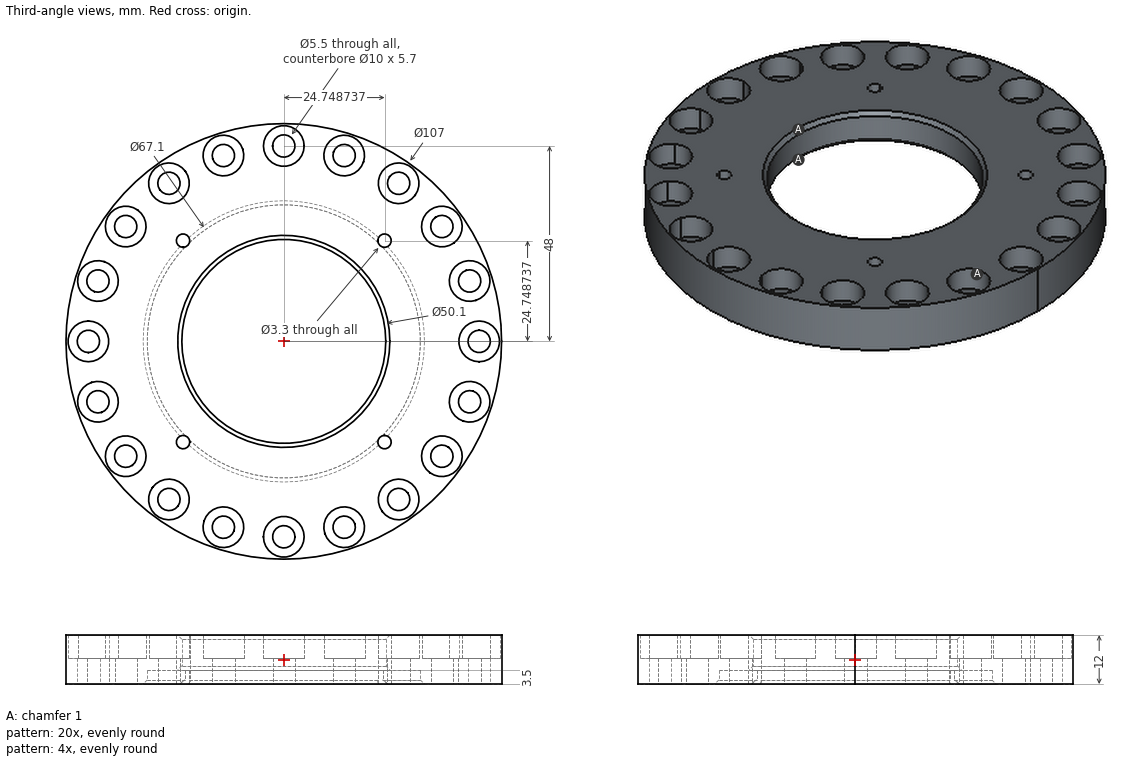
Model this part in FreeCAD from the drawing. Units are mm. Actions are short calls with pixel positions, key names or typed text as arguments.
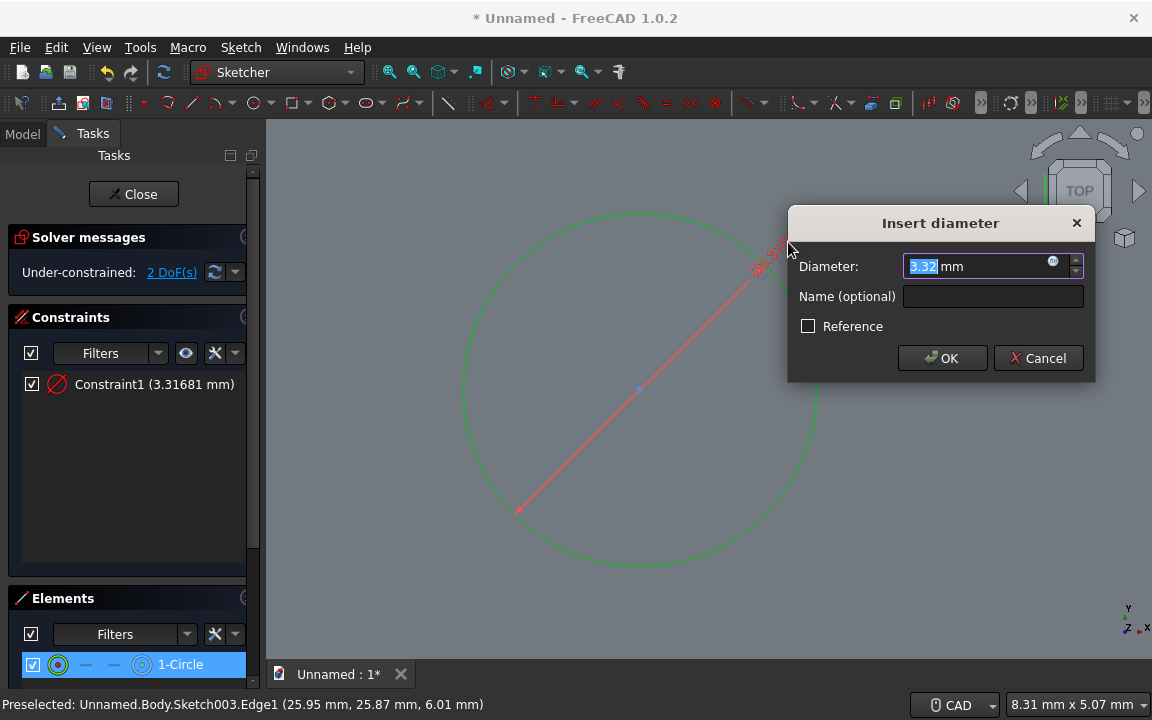
text(3.3)
key(Return)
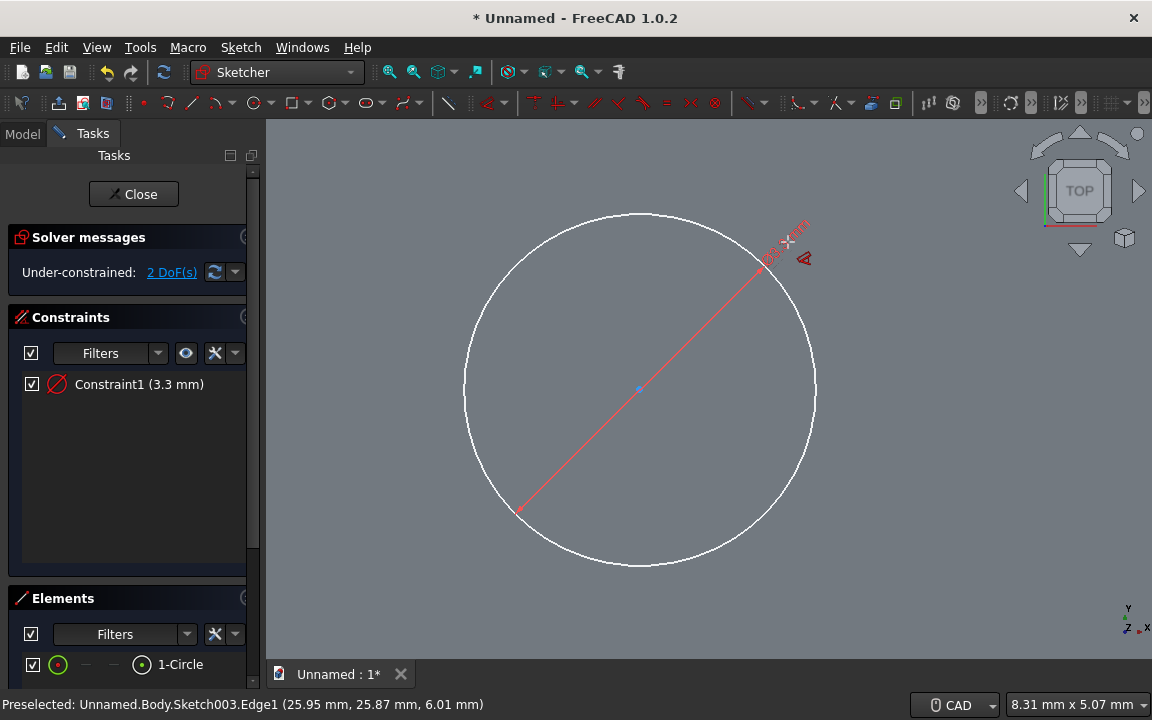
click(640, 390)
click(387, 356)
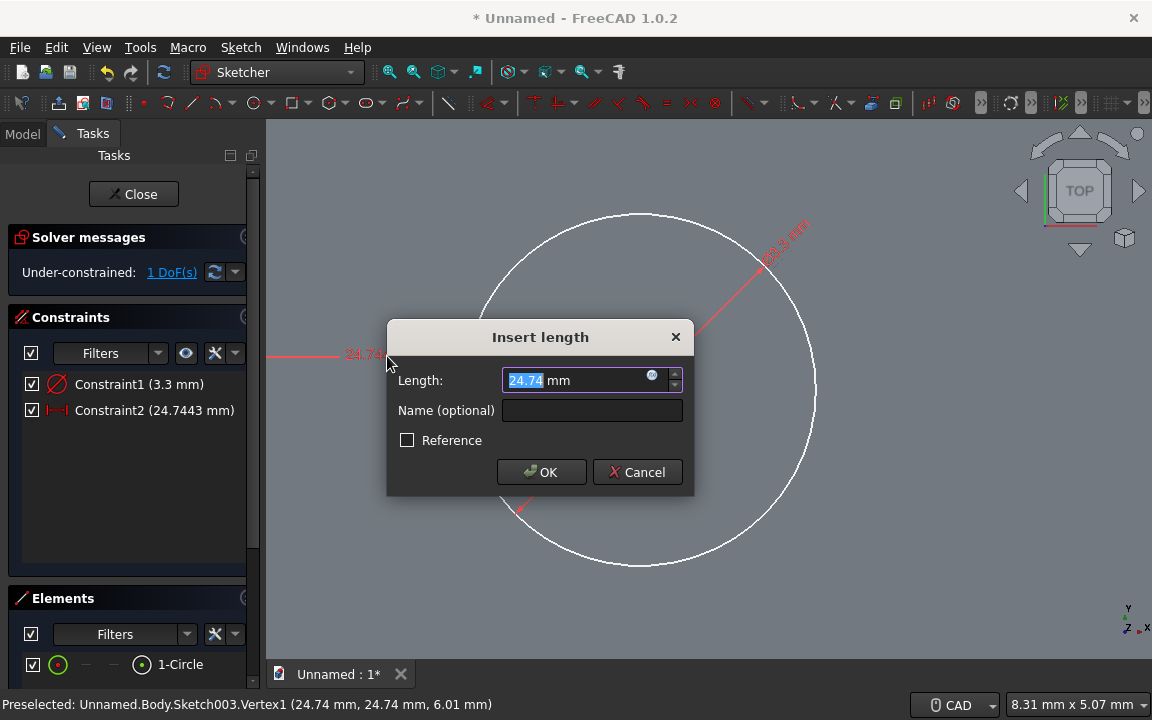
text(24.748737)
key(Return)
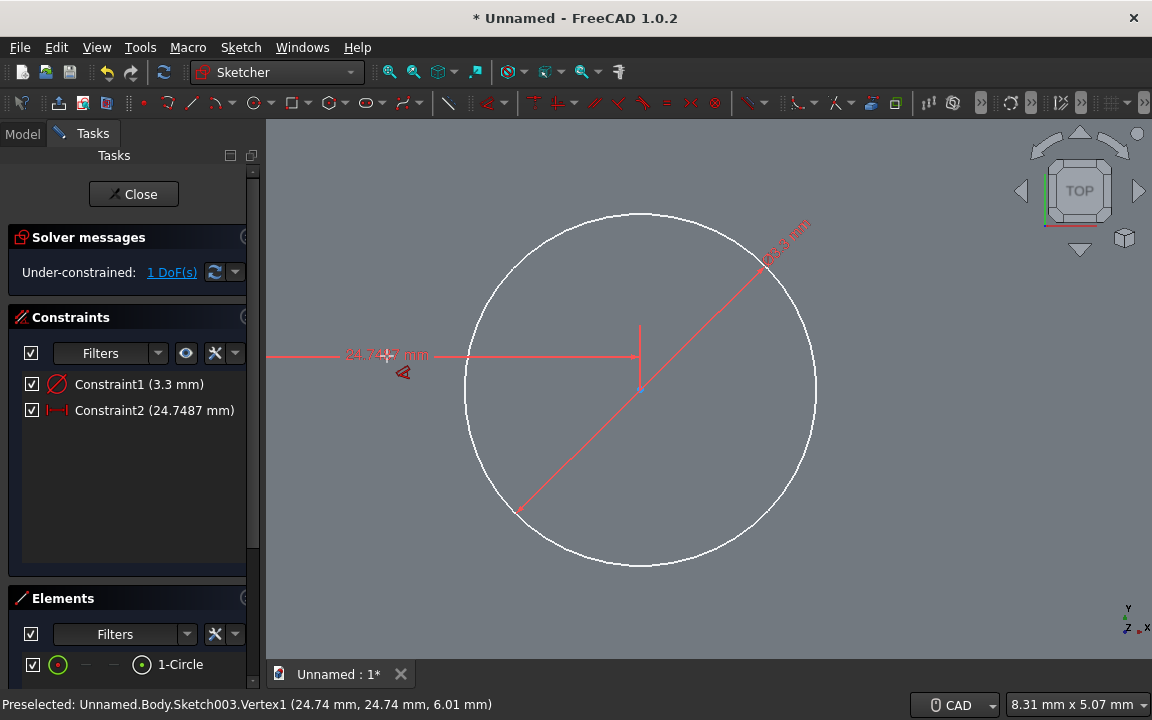
click(640, 390)
click(674, 511)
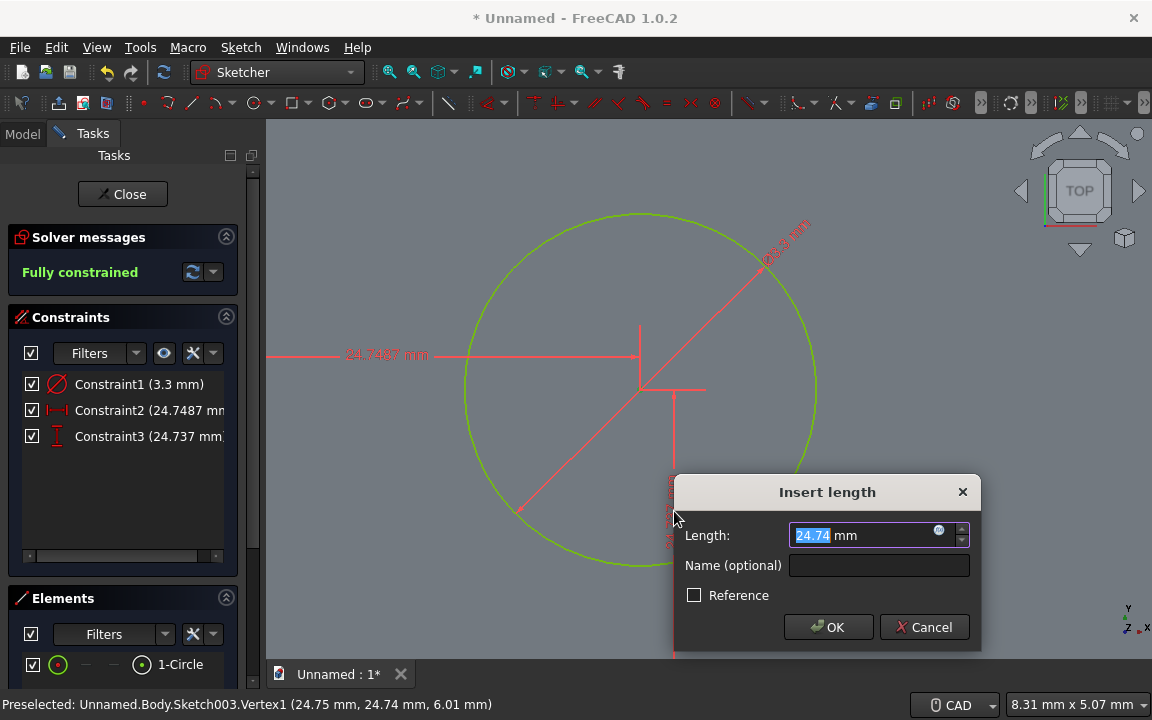
text(24.748737)
key(Return)
key(Escape)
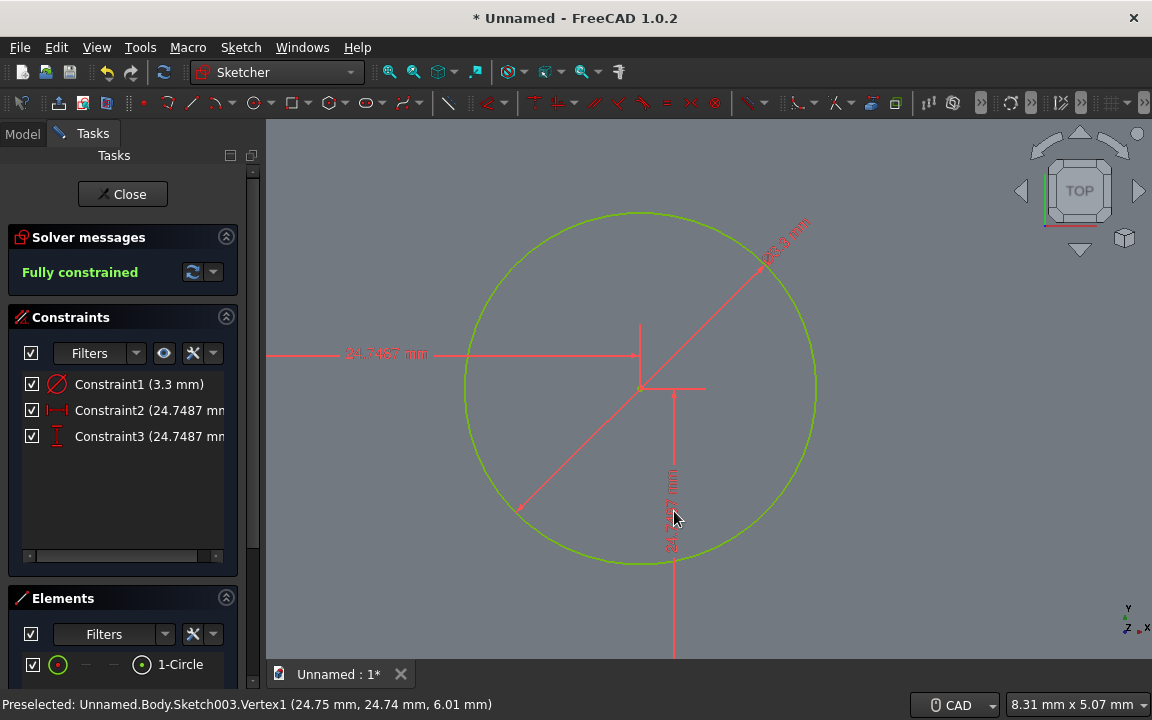
click(123, 194)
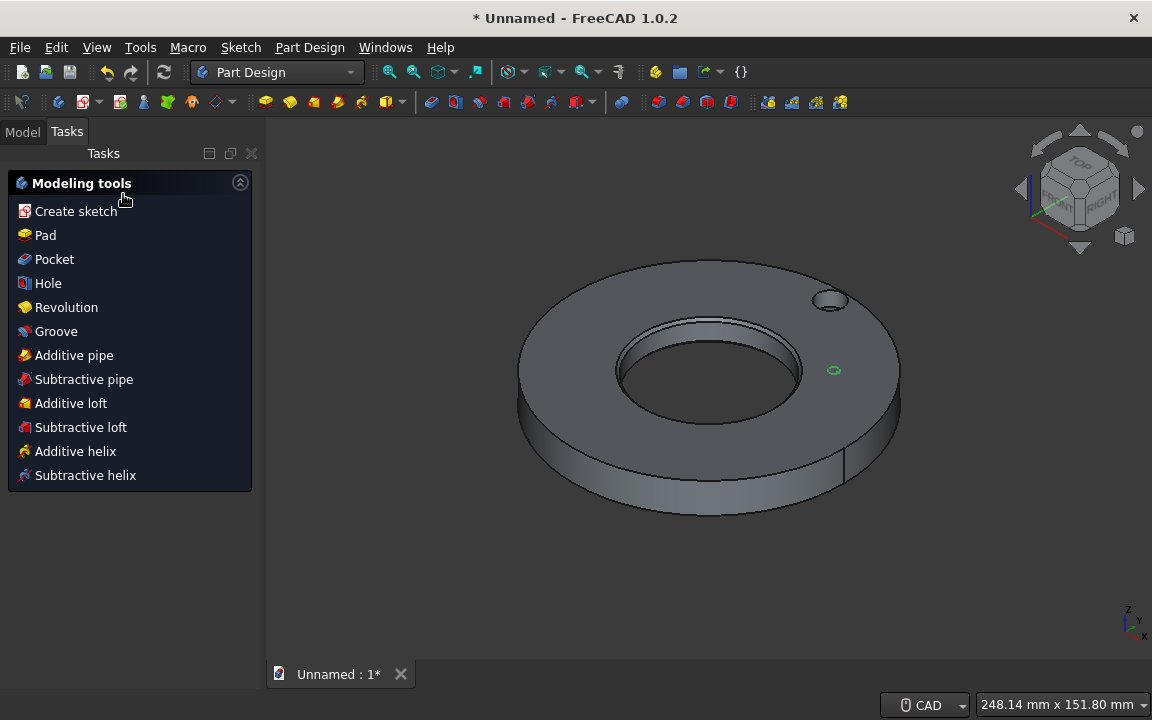
click(456, 102)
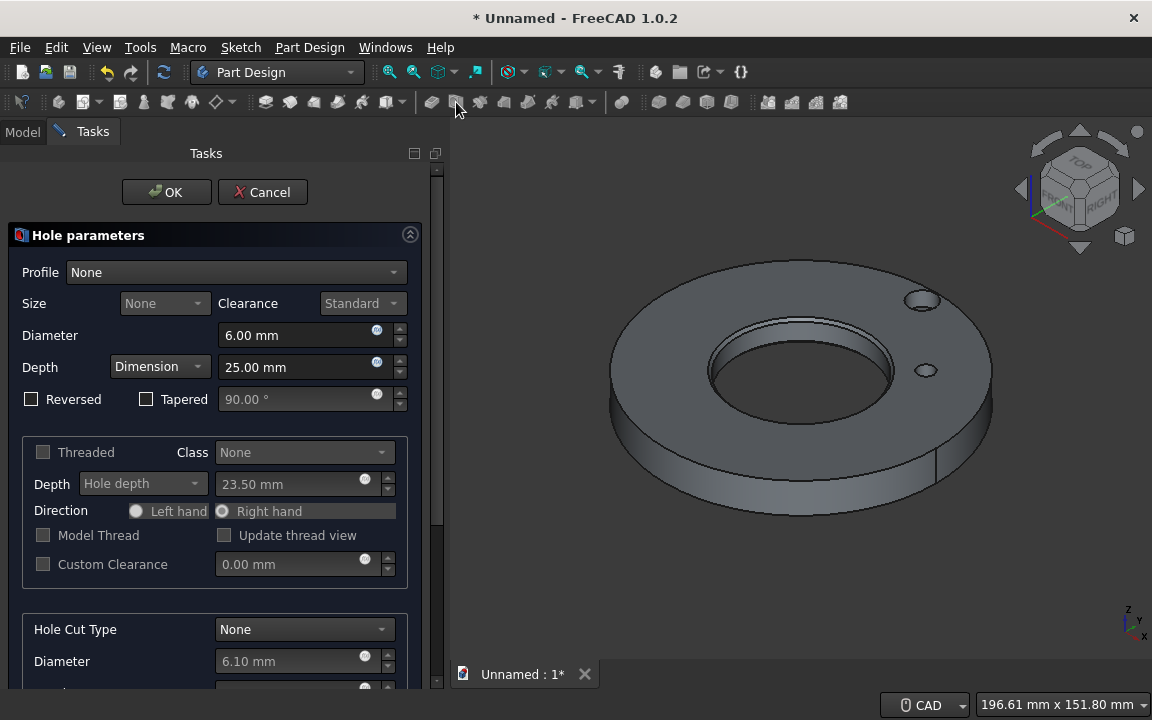
triple_click(305, 335)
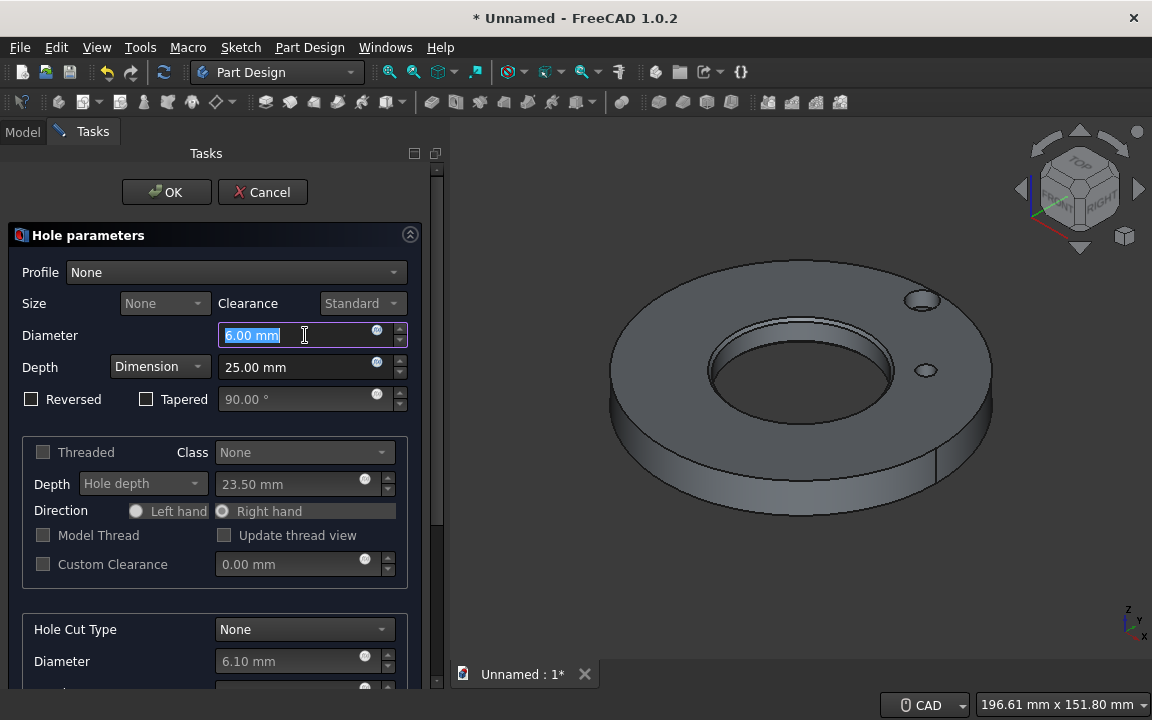
text(3.3)
key(Tab)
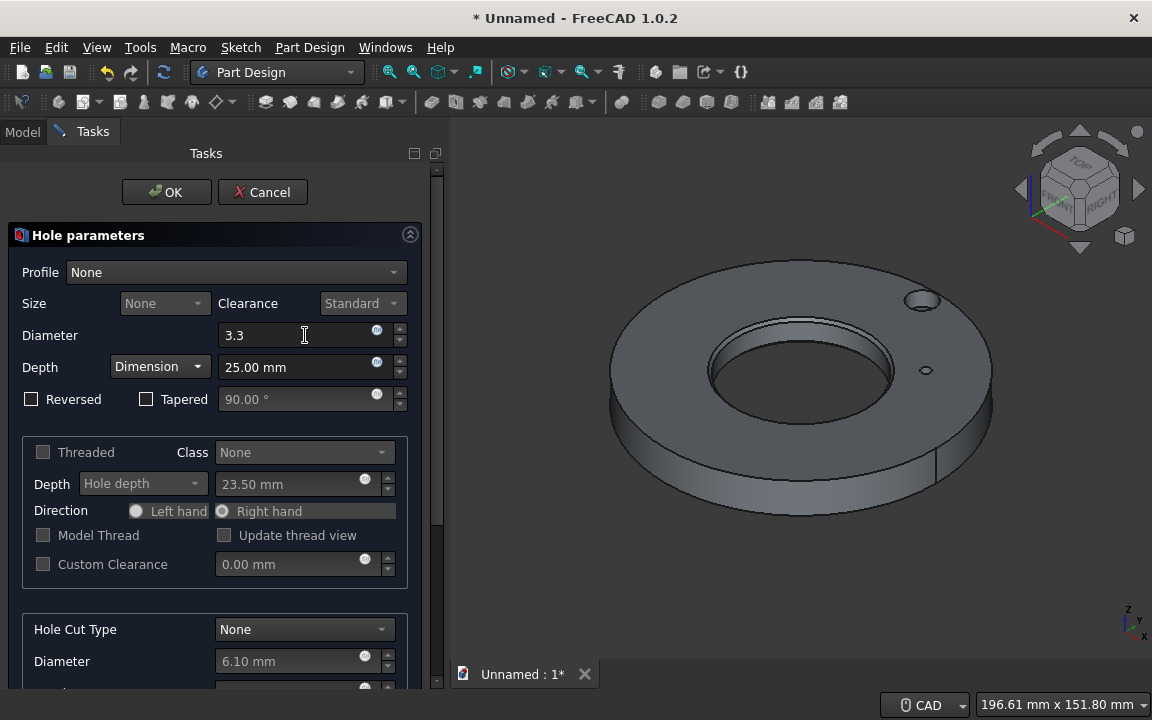
click(161, 366)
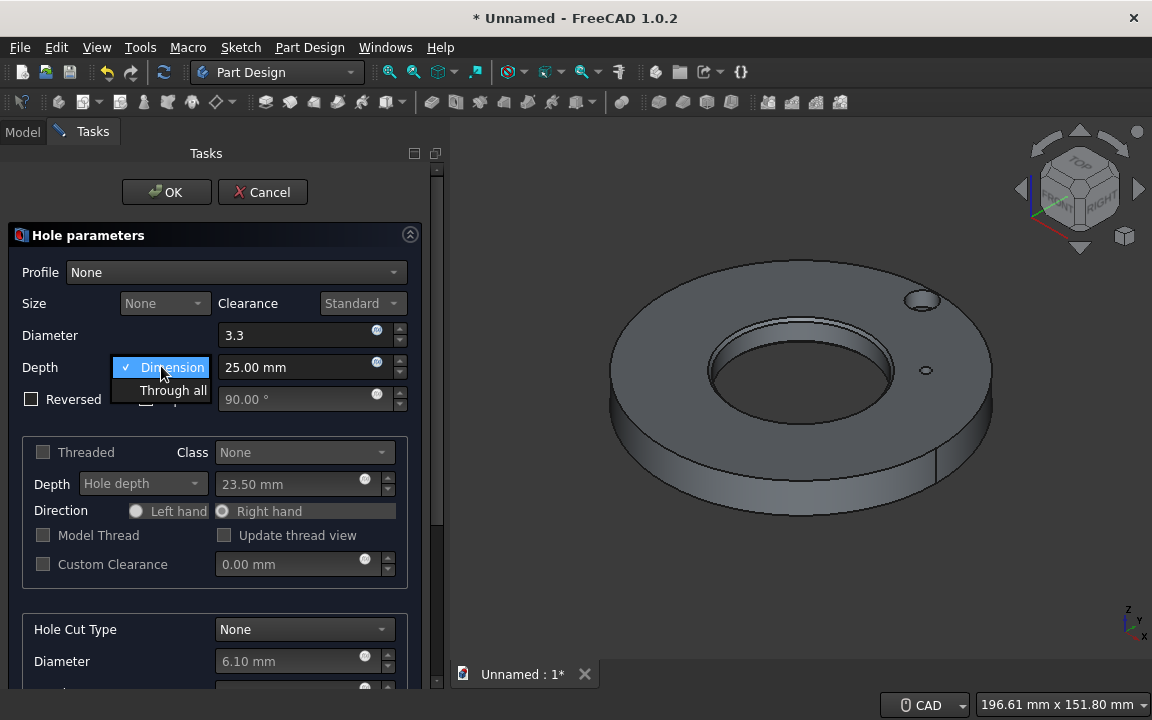
click(160, 390)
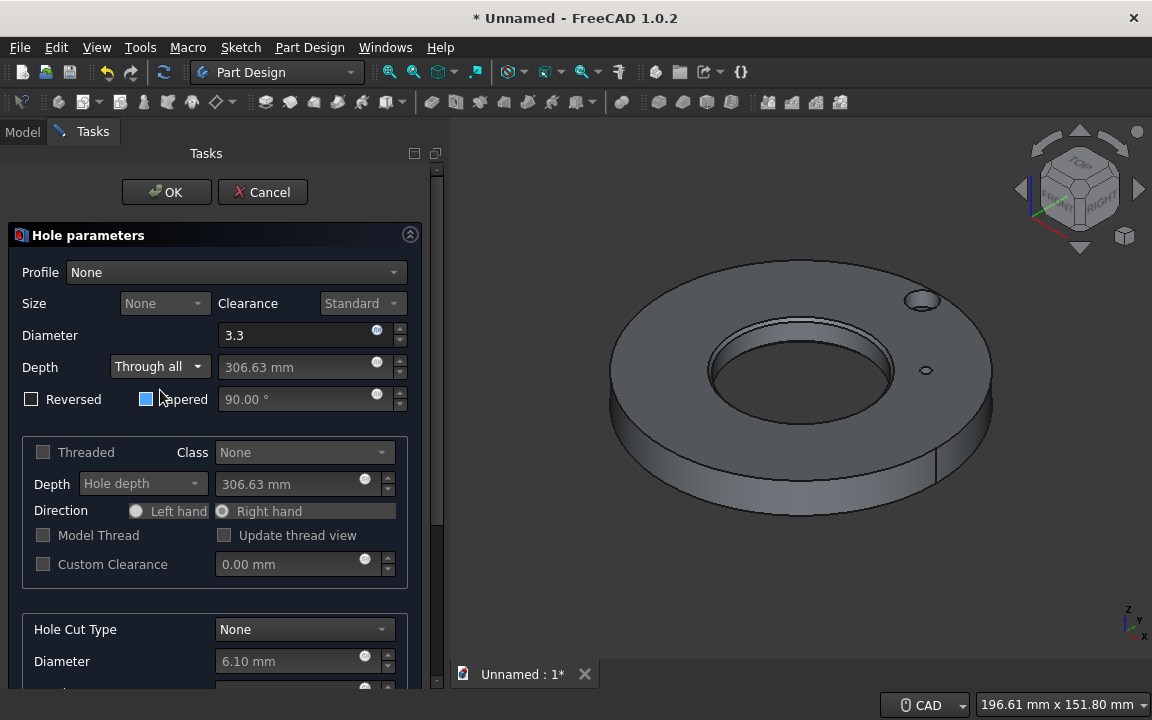
click(167, 192)